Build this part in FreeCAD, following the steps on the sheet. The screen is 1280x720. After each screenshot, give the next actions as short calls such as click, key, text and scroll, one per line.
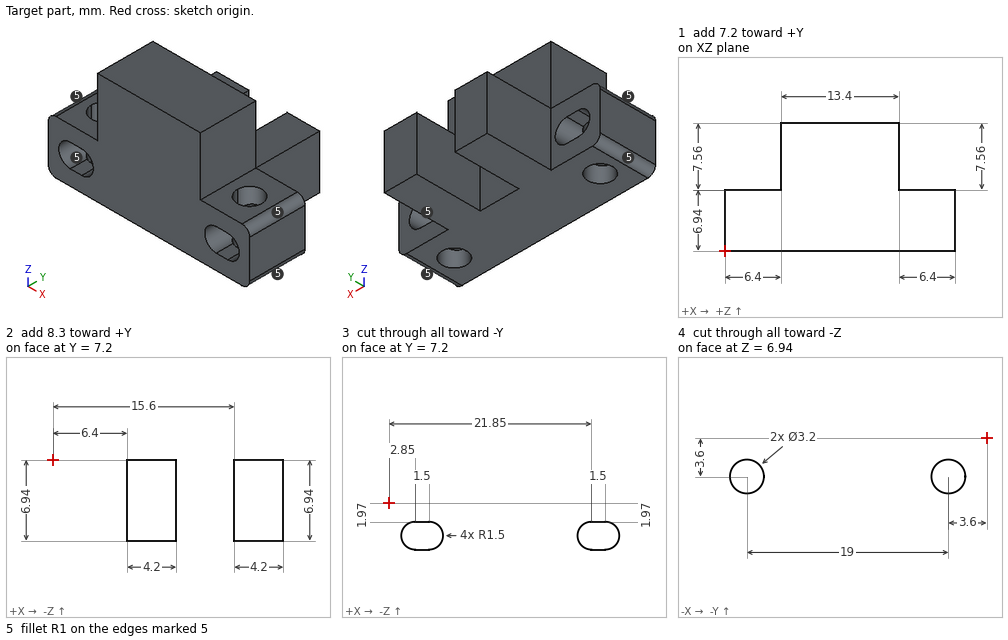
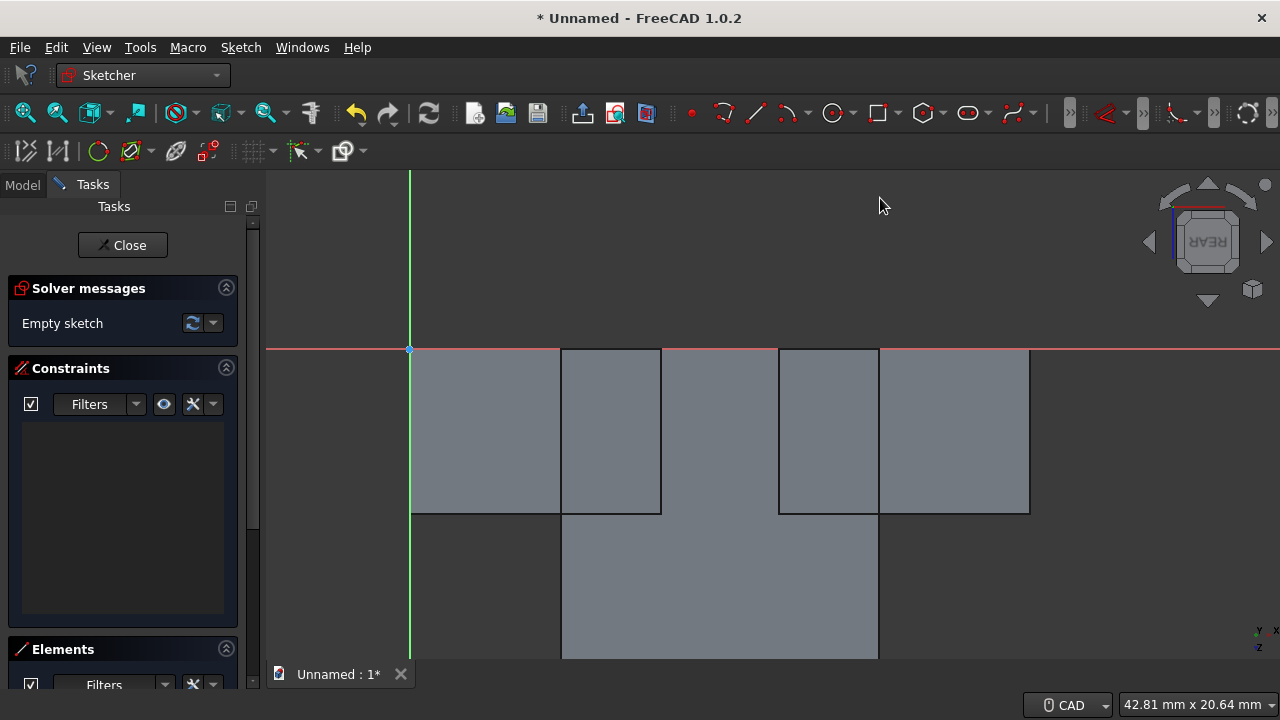
click(968, 114)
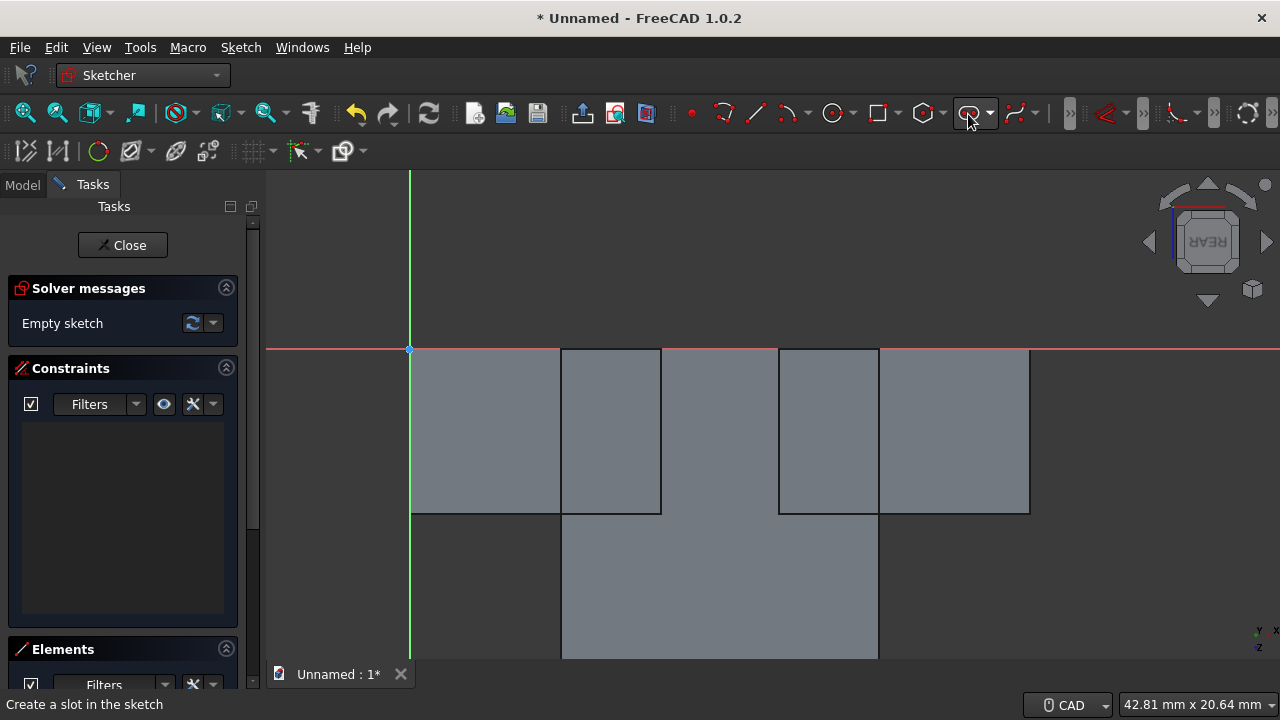
click(477, 431)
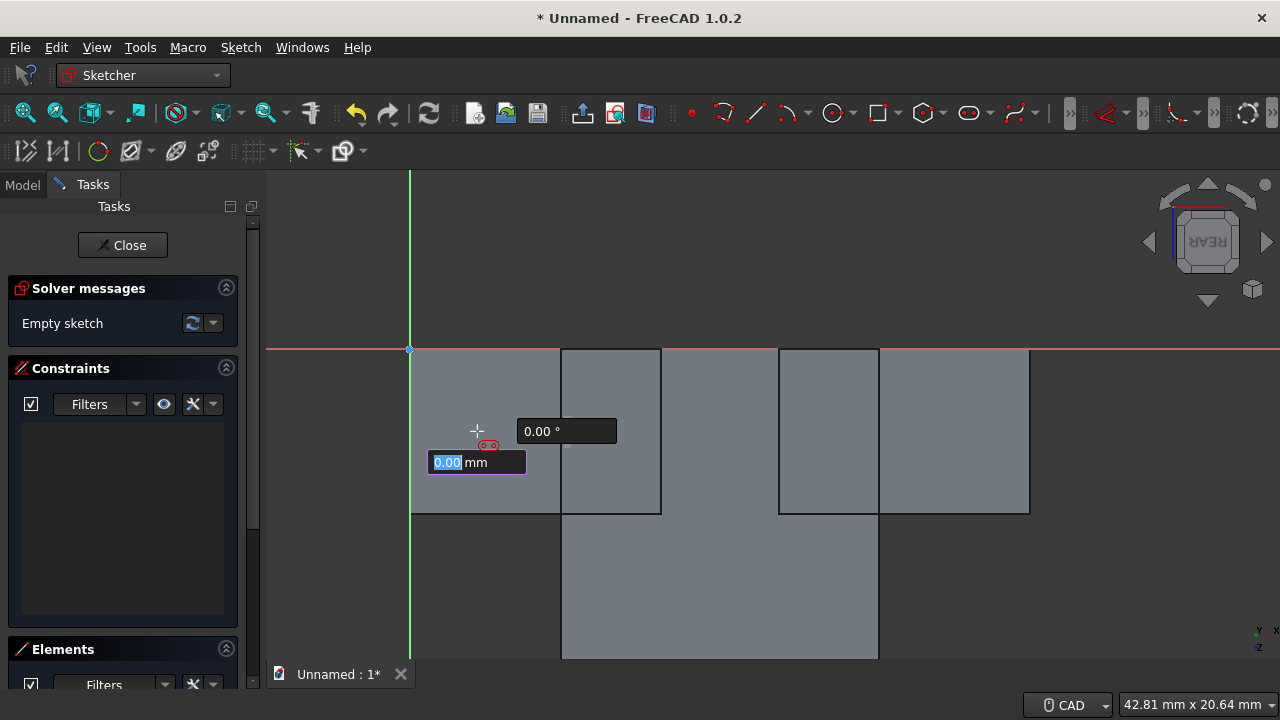
click(513, 431)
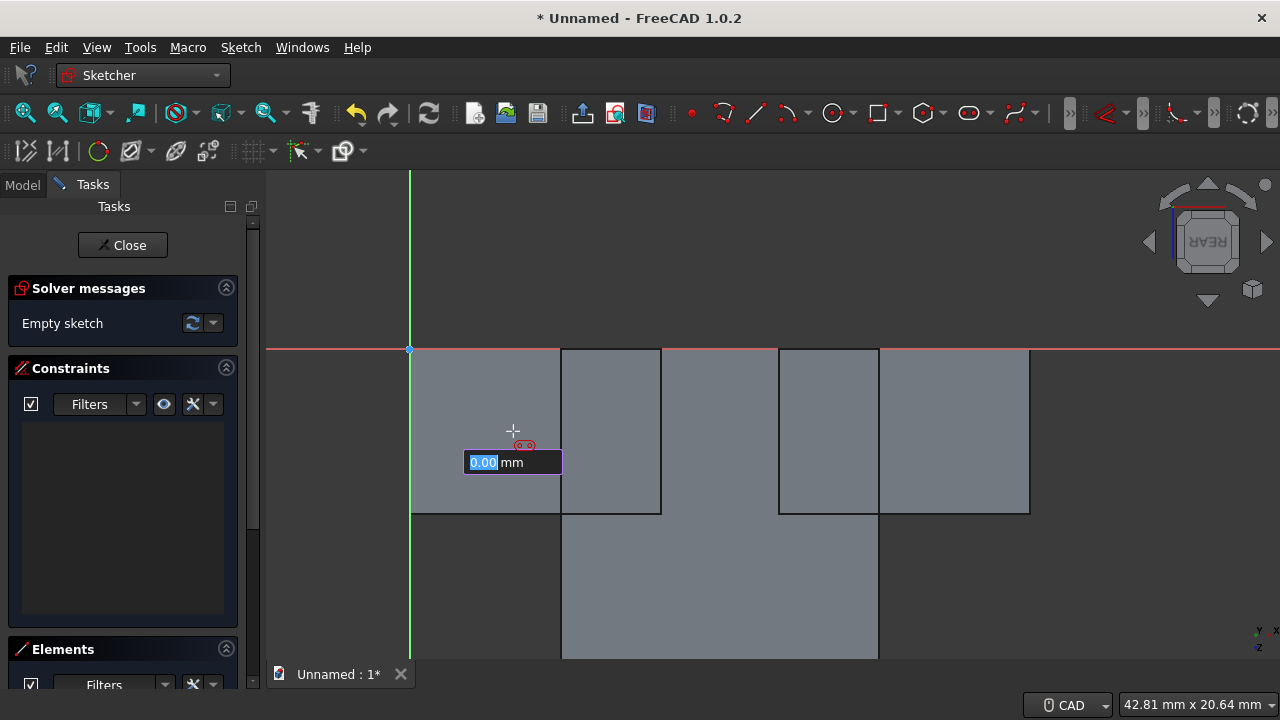
click(495, 396)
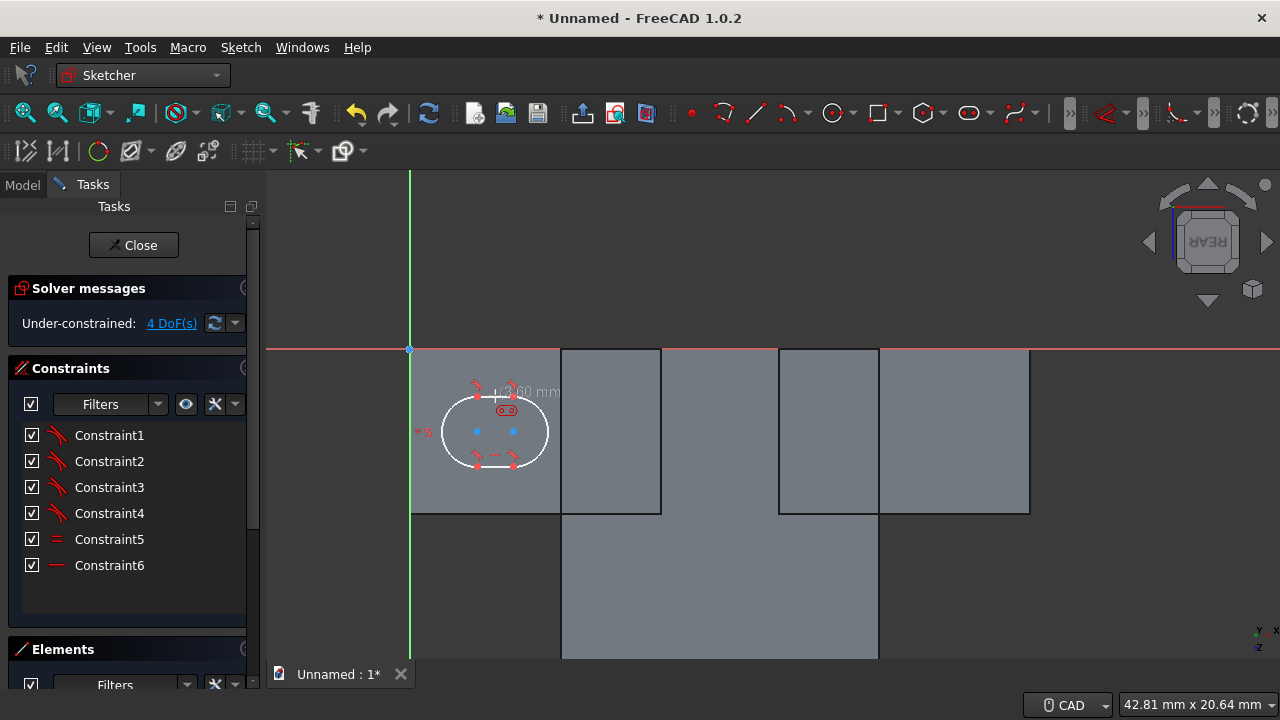
click(927, 431)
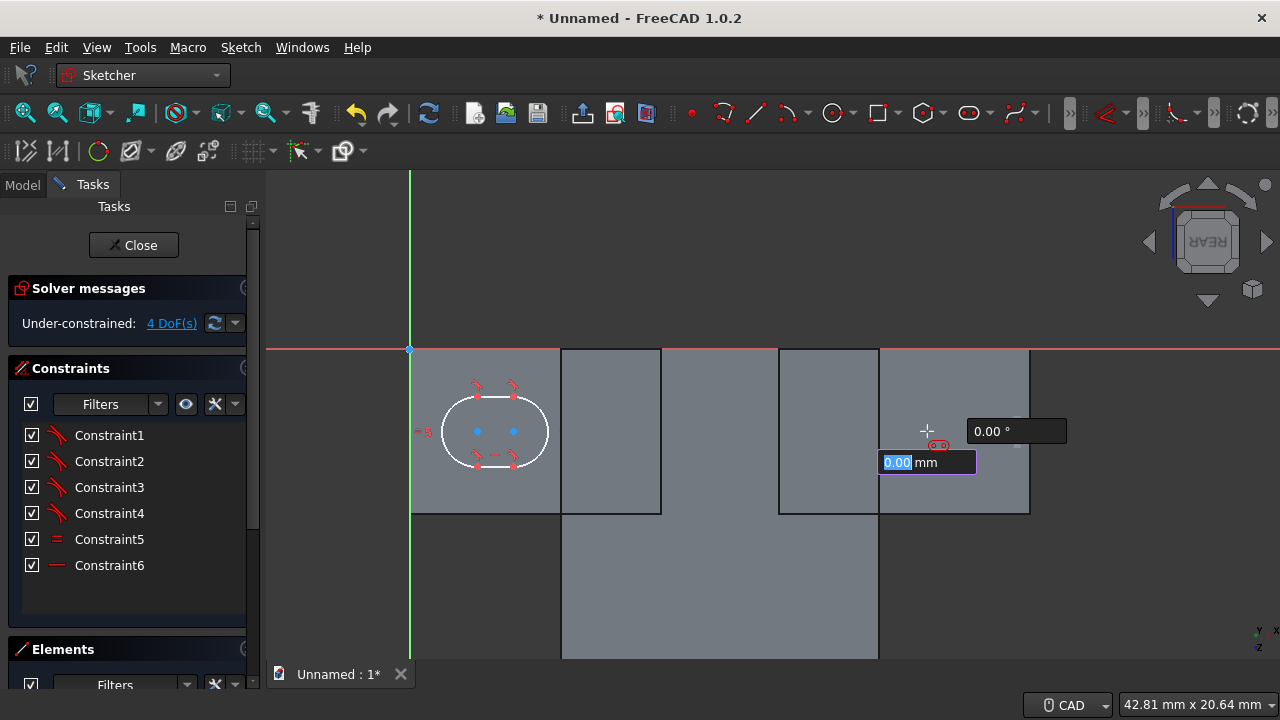
click(963, 431)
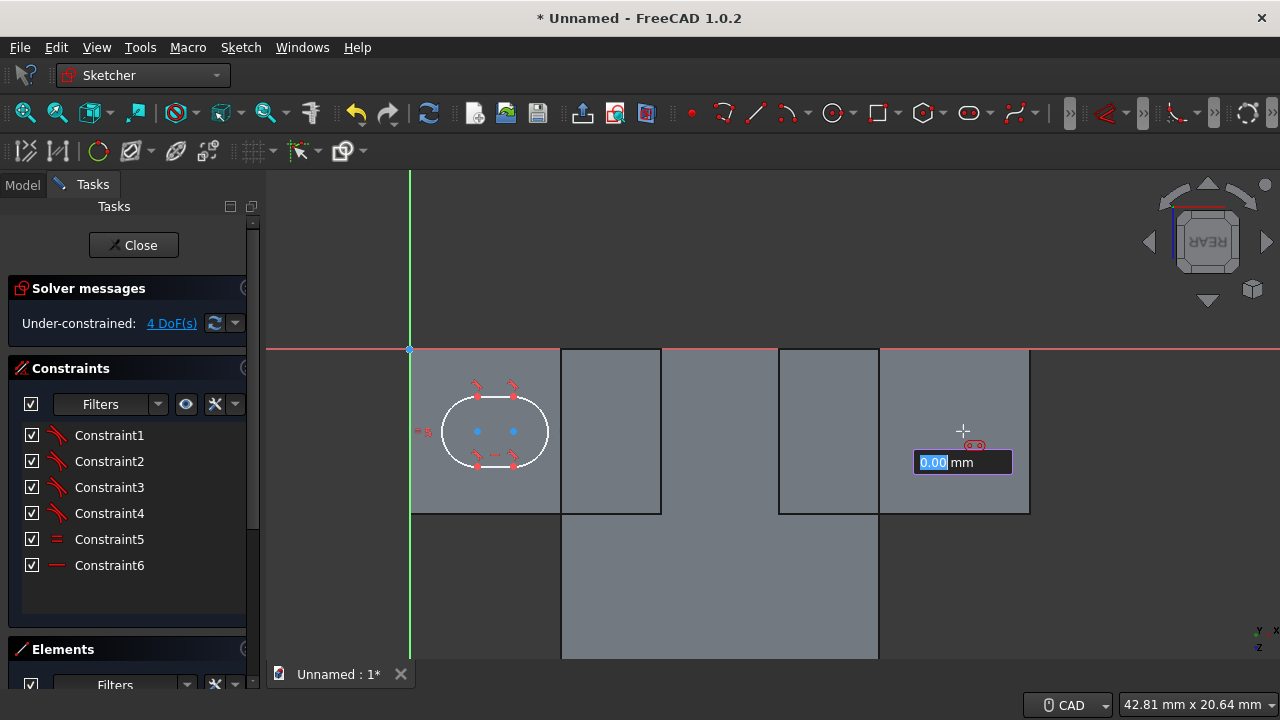
click(945, 467)
key(Escape)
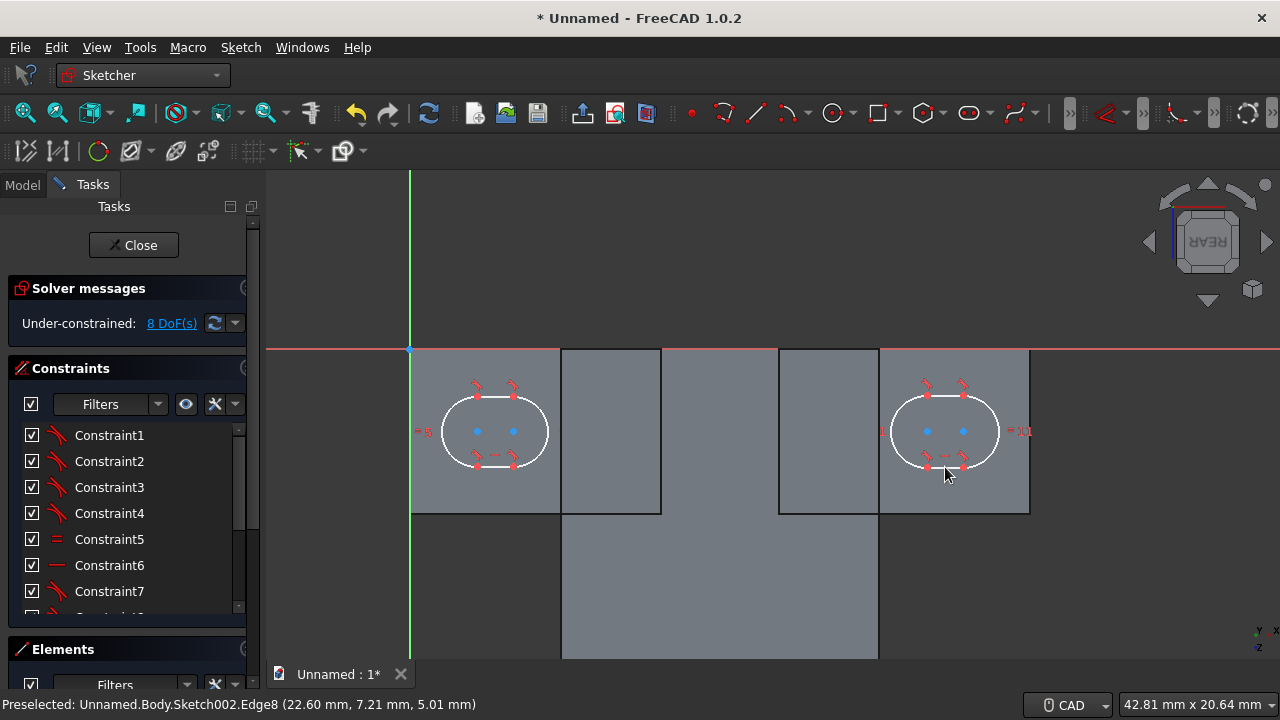
click(449, 411)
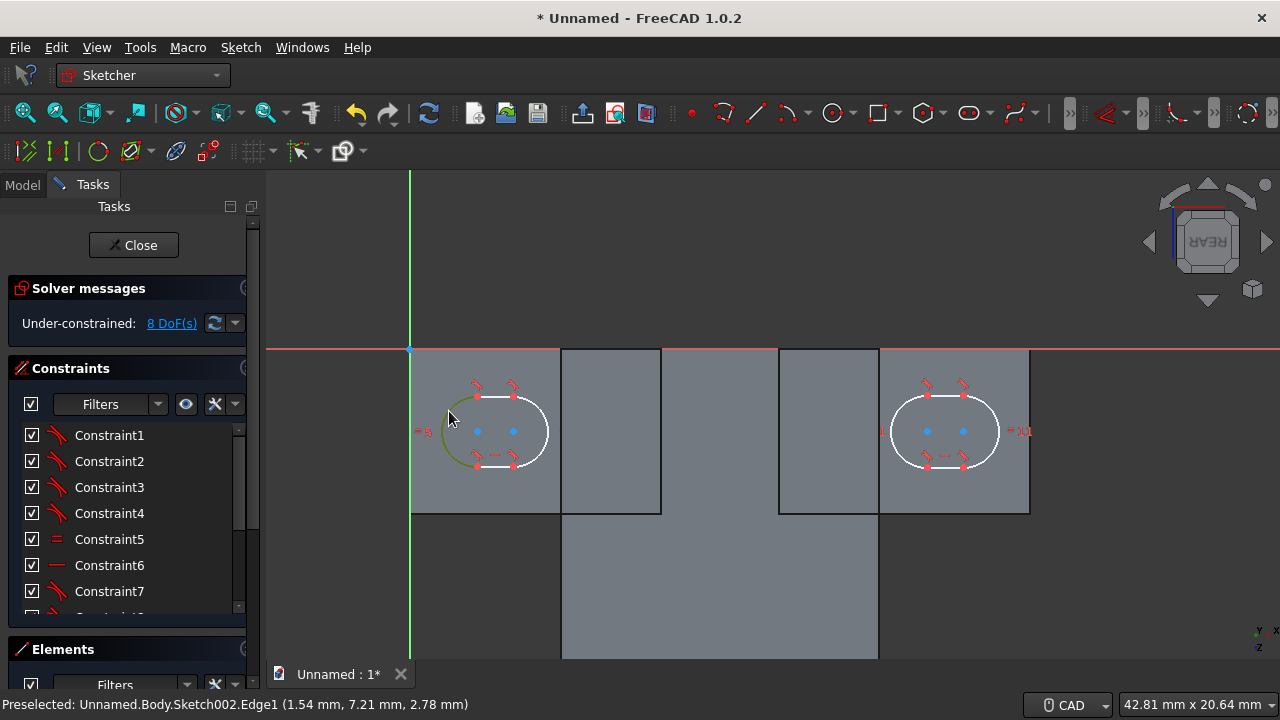
click(898, 411)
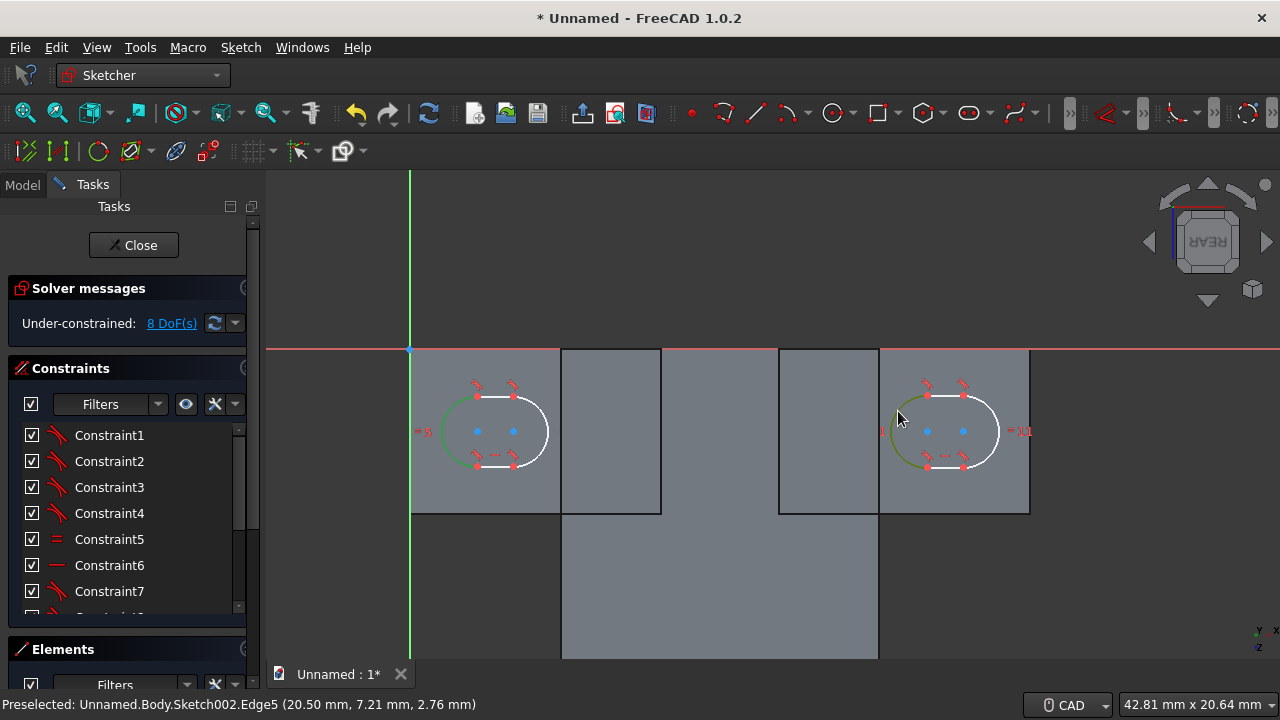
key(e)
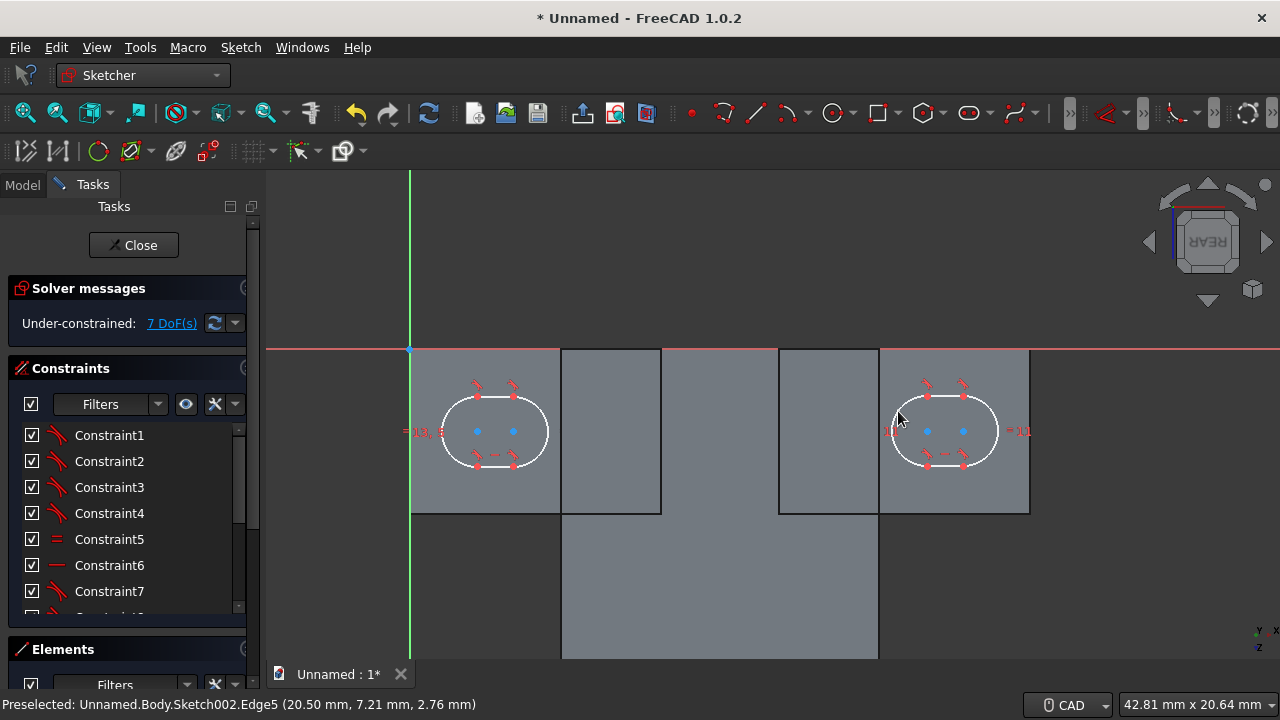
click(1106, 114)